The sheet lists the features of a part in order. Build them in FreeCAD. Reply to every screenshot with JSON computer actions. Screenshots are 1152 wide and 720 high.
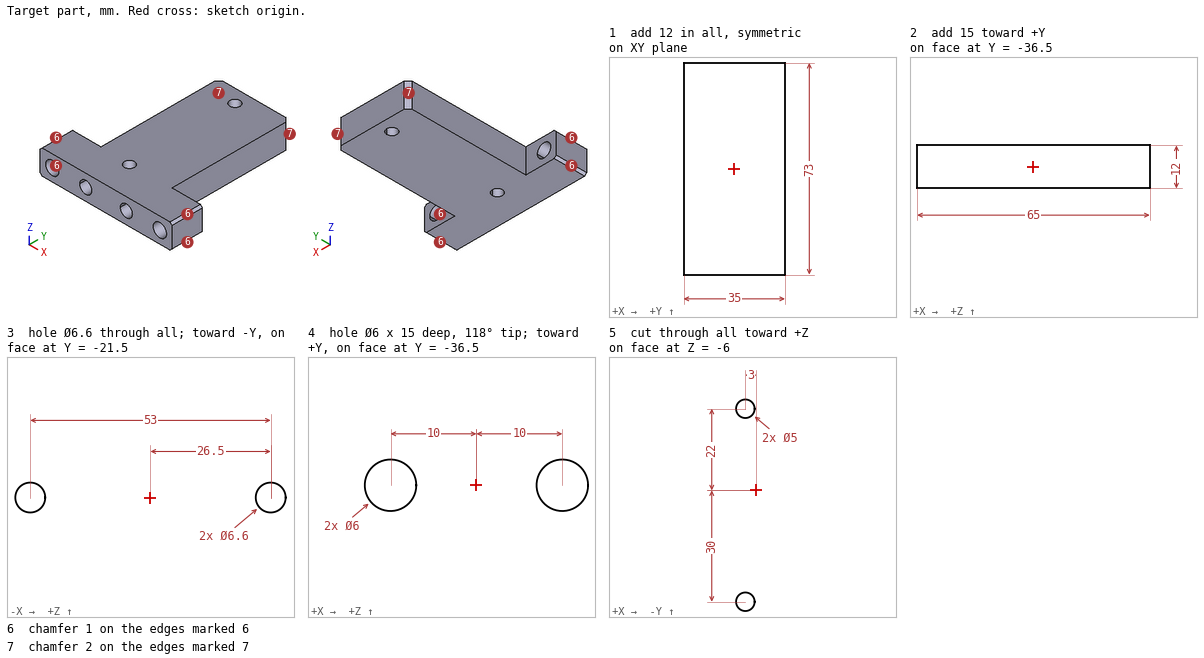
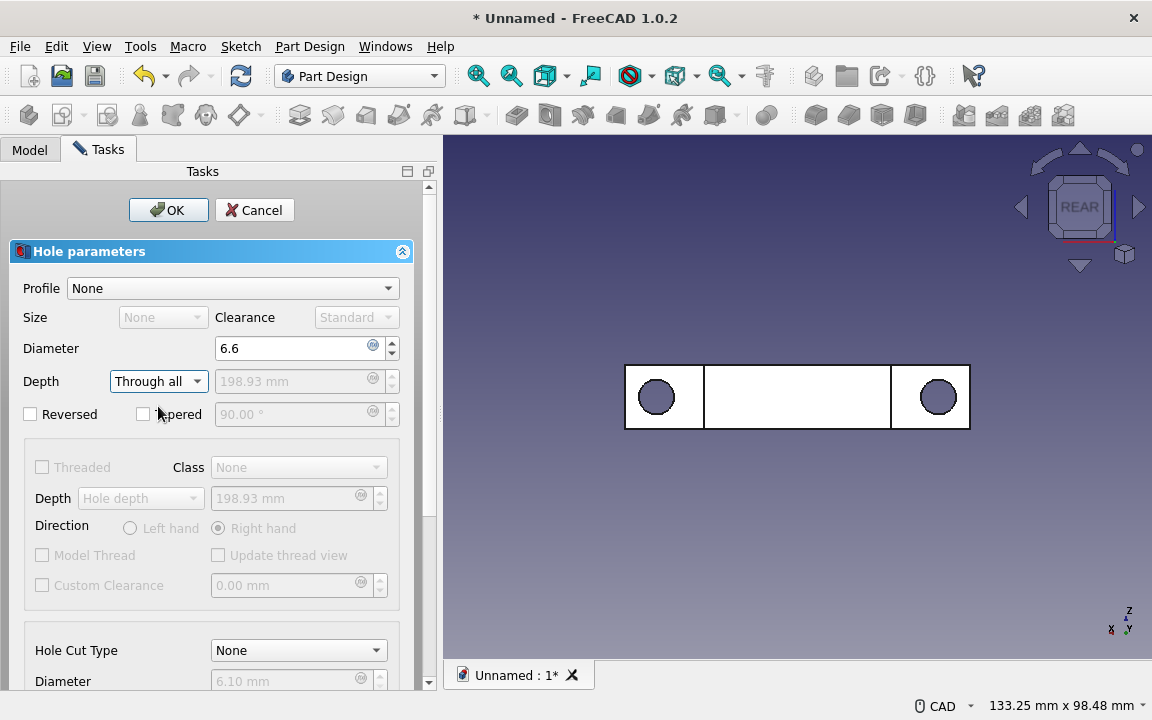
{"action": "left_click", "coordinate": [169, 210]}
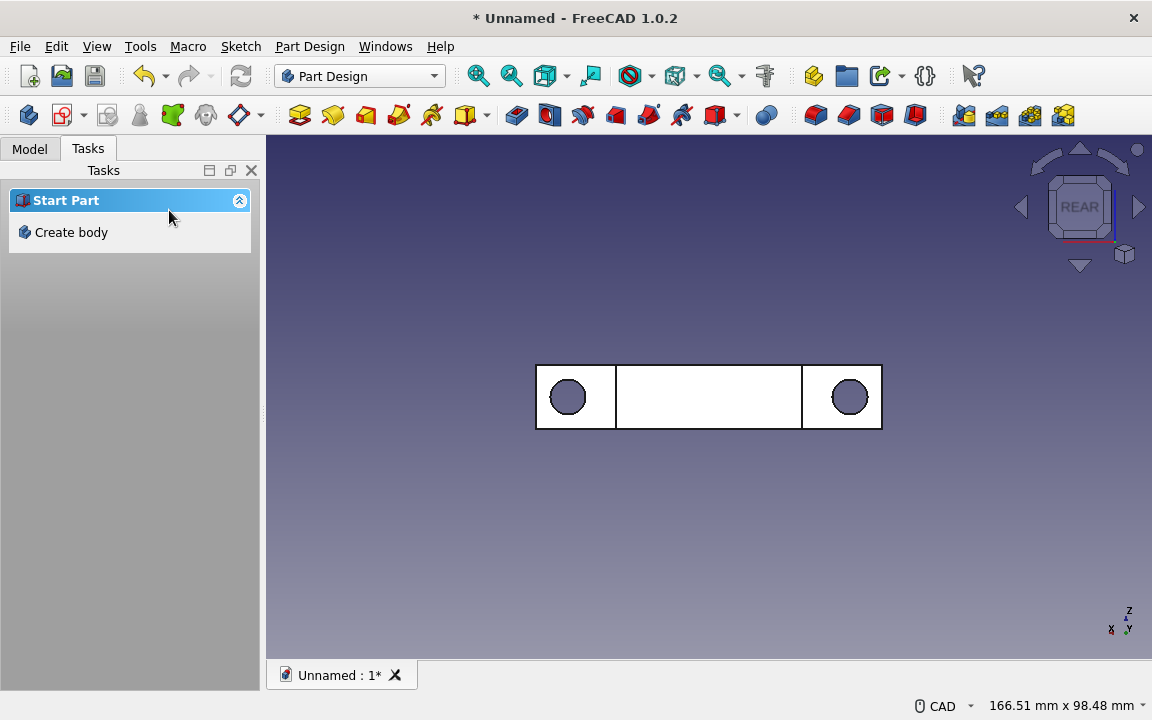
{"action": "left_click", "coordinate": [479, 76]}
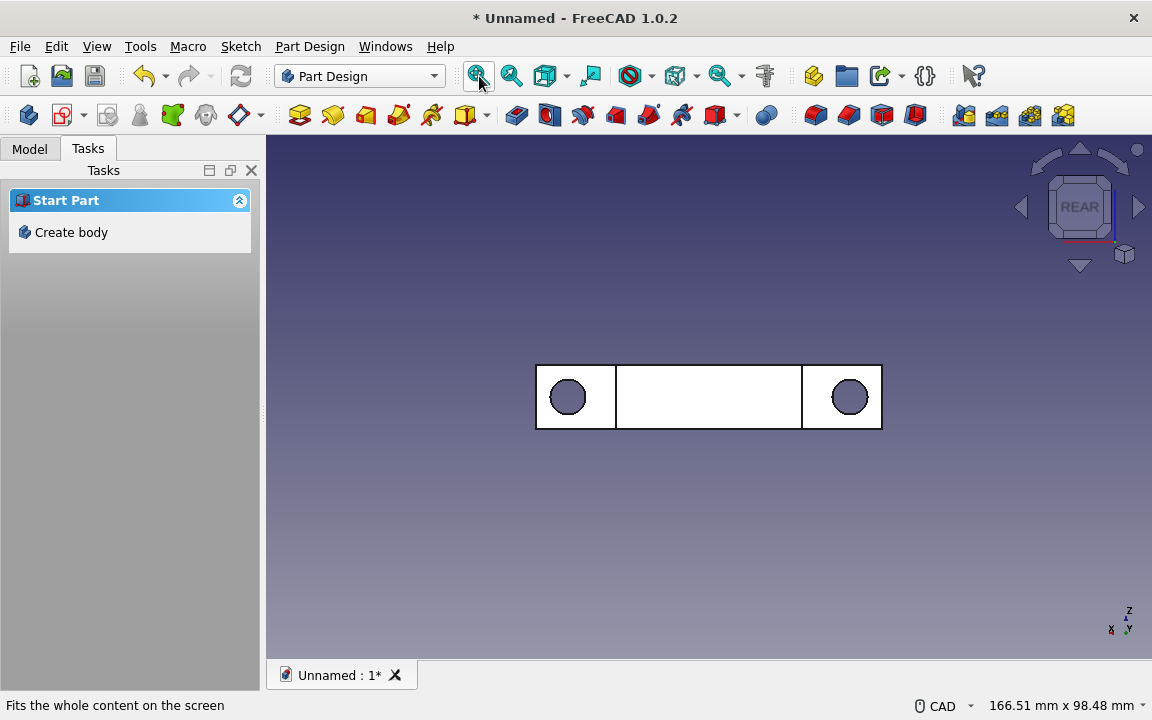
{"action": "key", "text": "0"}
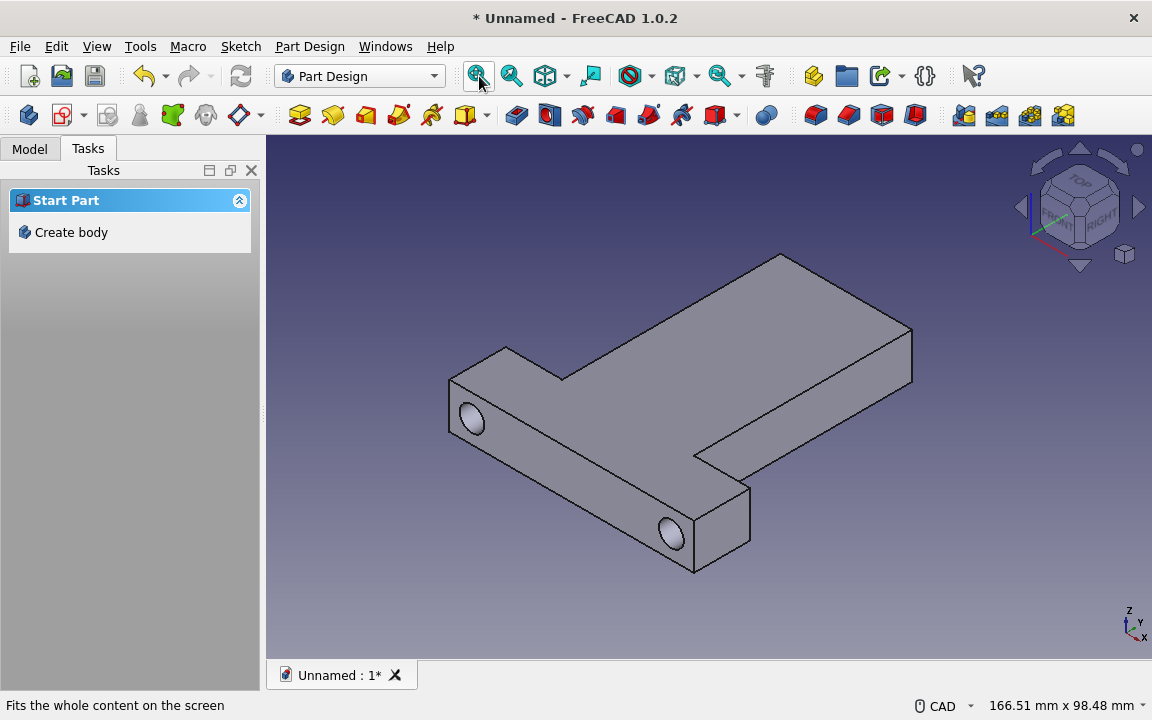
{"action": "left_click", "coordinate": [607, 495]}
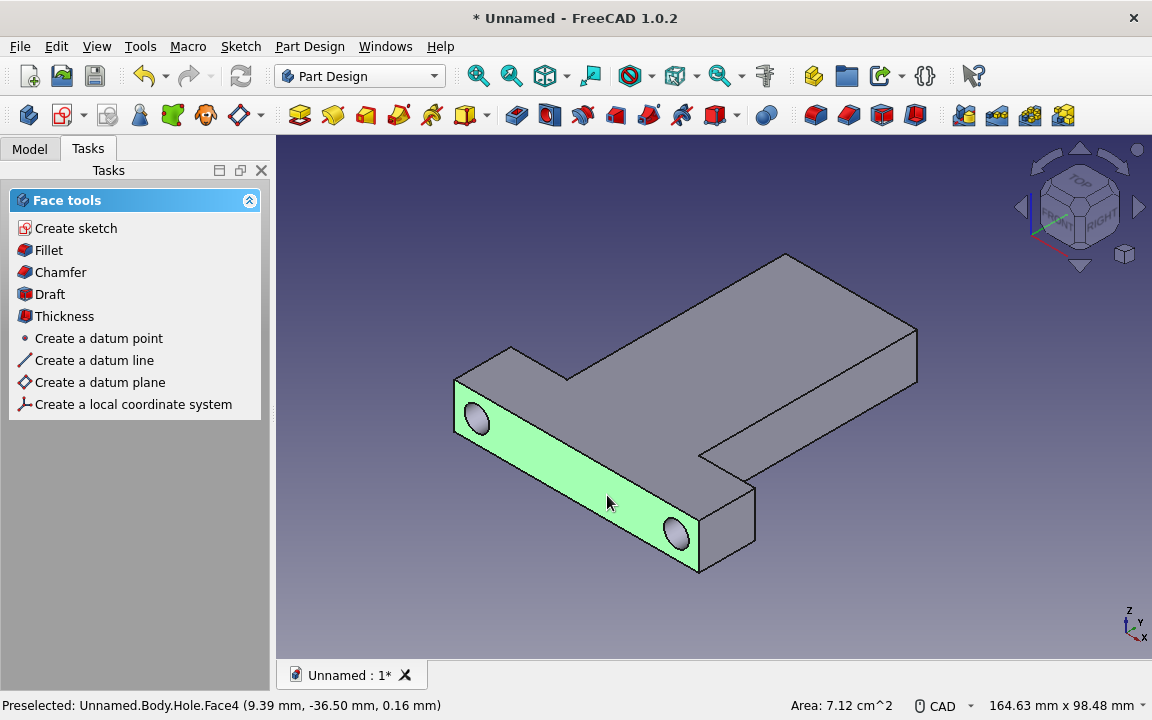
{"action": "left_click", "coordinate": [62, 116]}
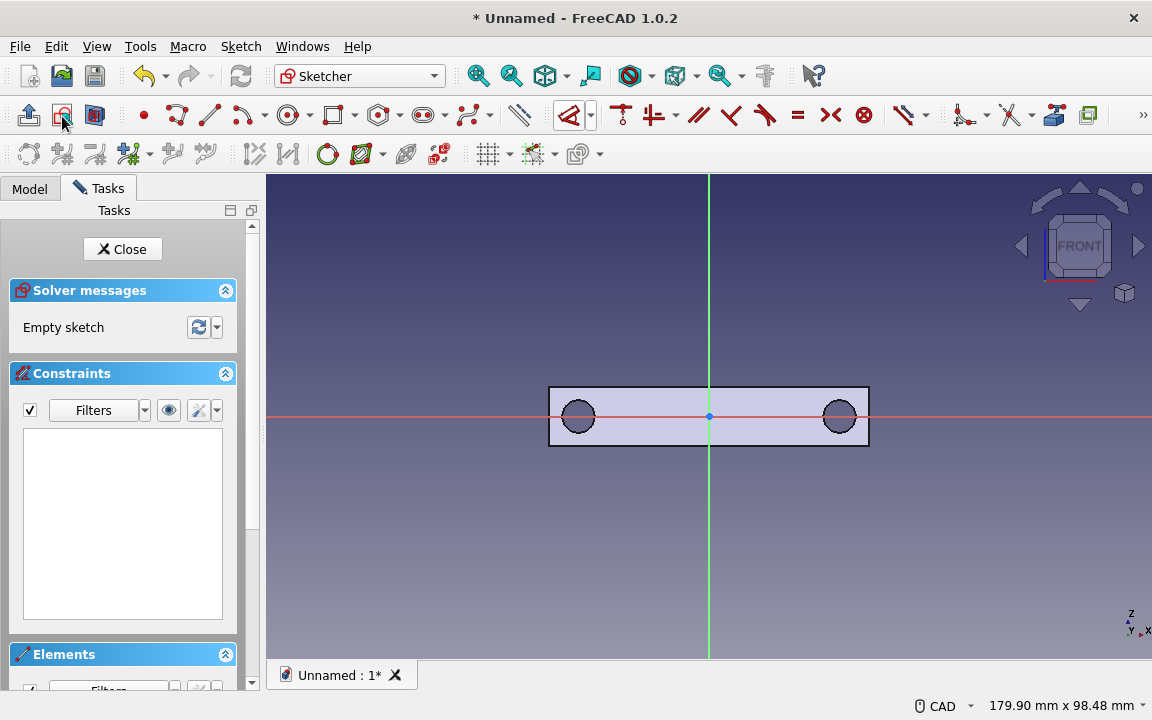
{"action": "scroll", "coordinate": [731, 417], "scroll_direction": "up", "scroll_amount": 7}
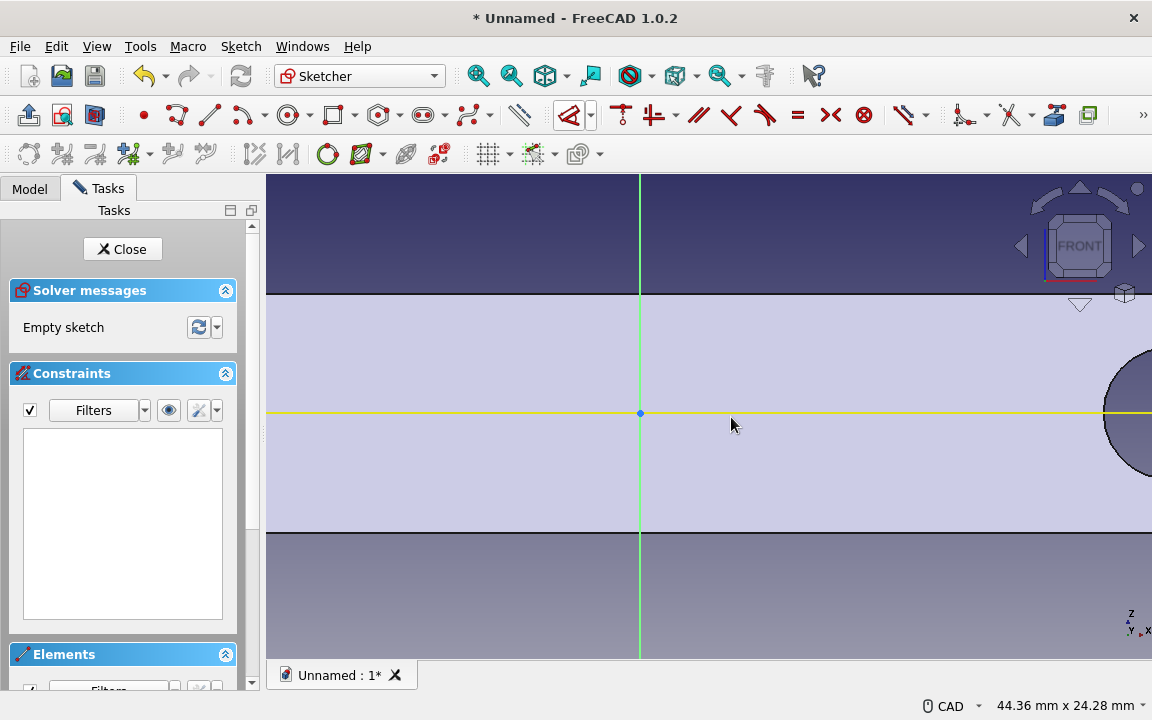
{"action": "left_click", "coordinate": [288, 116]}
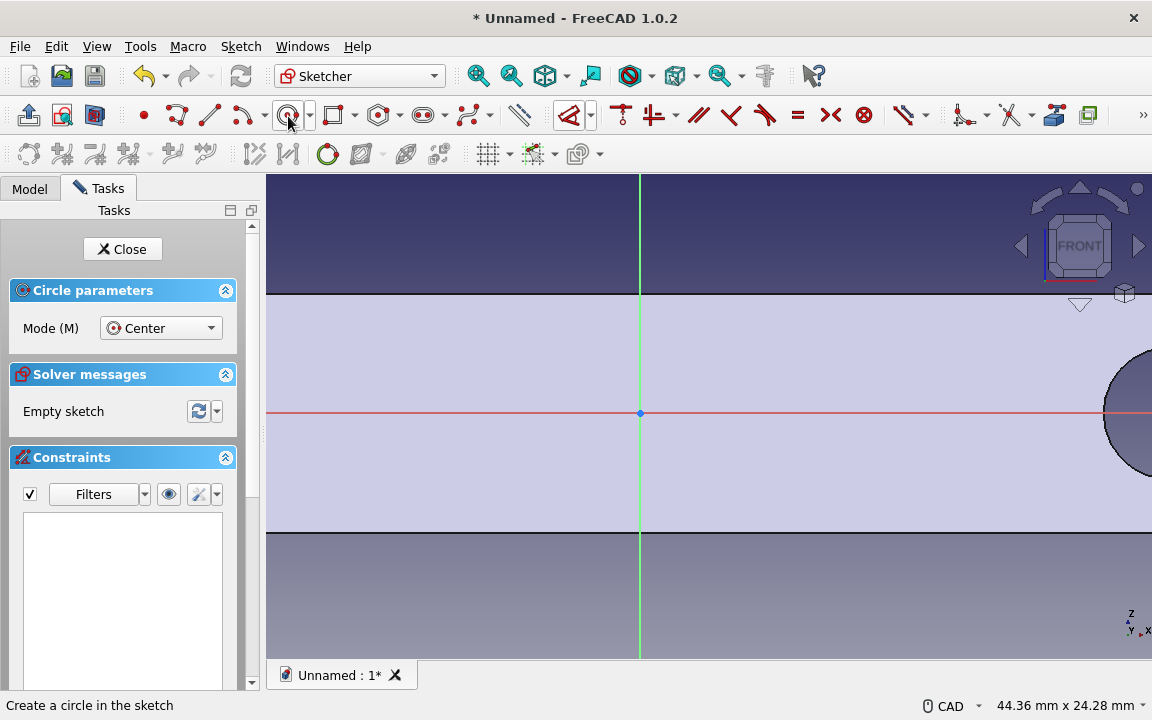
{"action": "left_click", "coordinate": [440, 413]}
{"action": "mouse_move", "coordinate": [483, 371]}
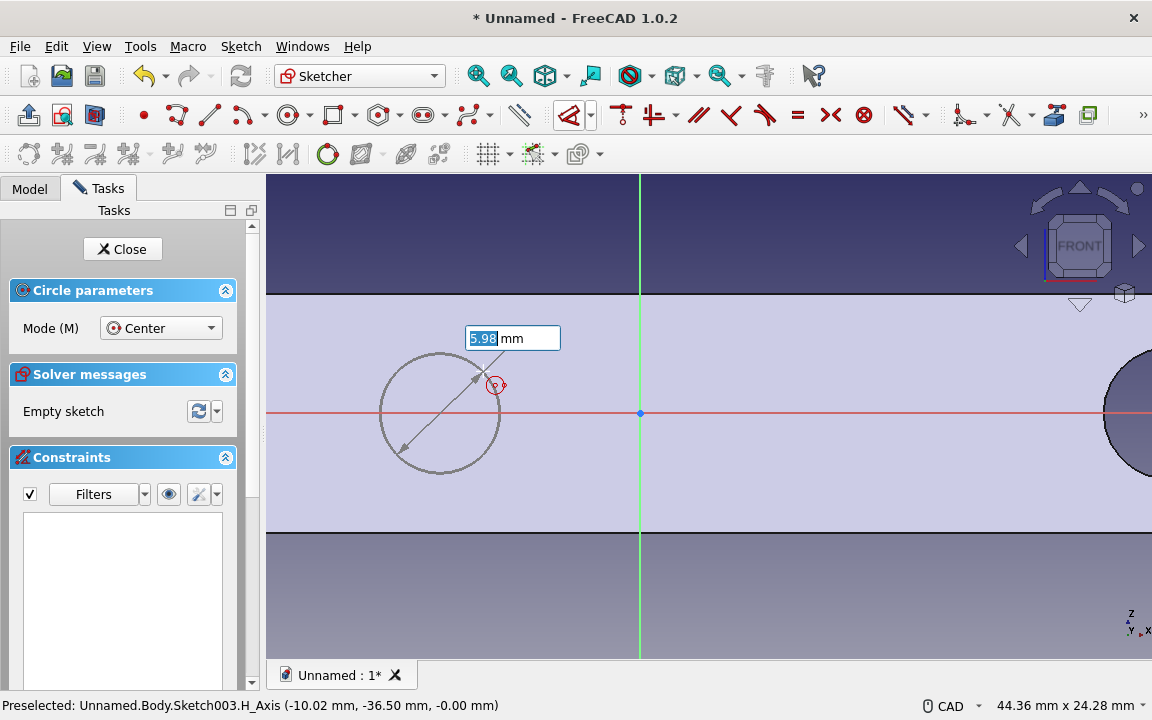
{"action": "type", "text": "6"}
{"action": "key", "text": "Return"}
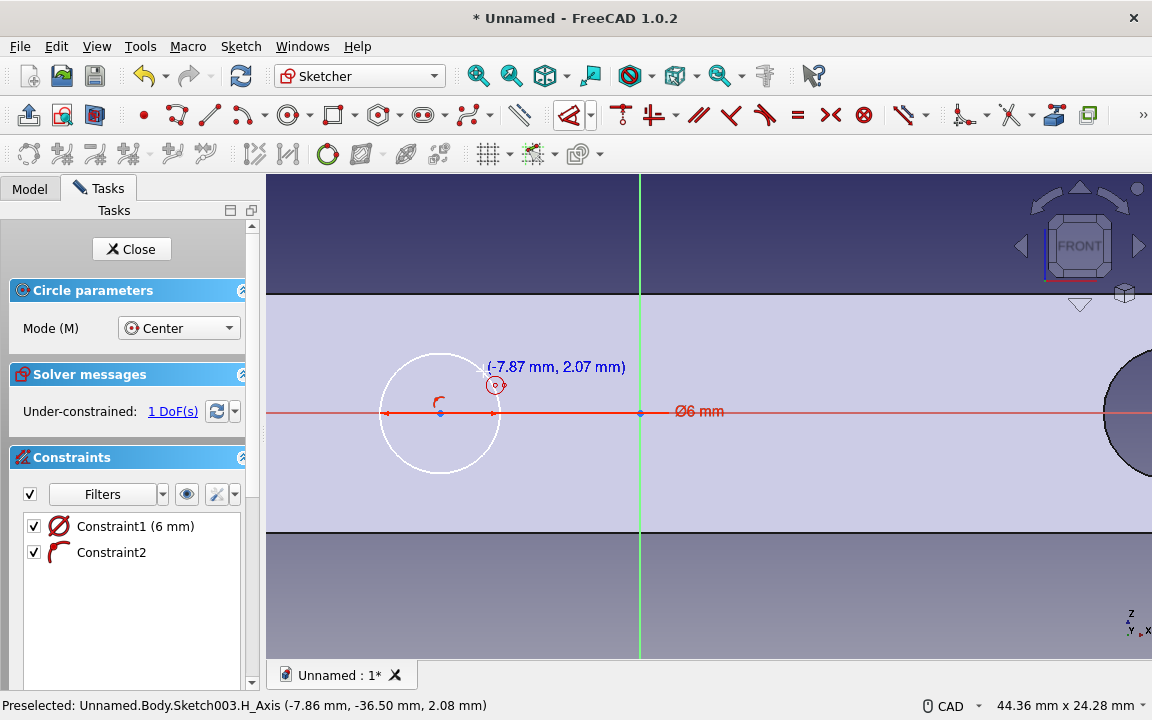
{"action": "left_click", "coordinate": [840, 413]}
{"action": "mouse_move", "coordinate": [882, 371]}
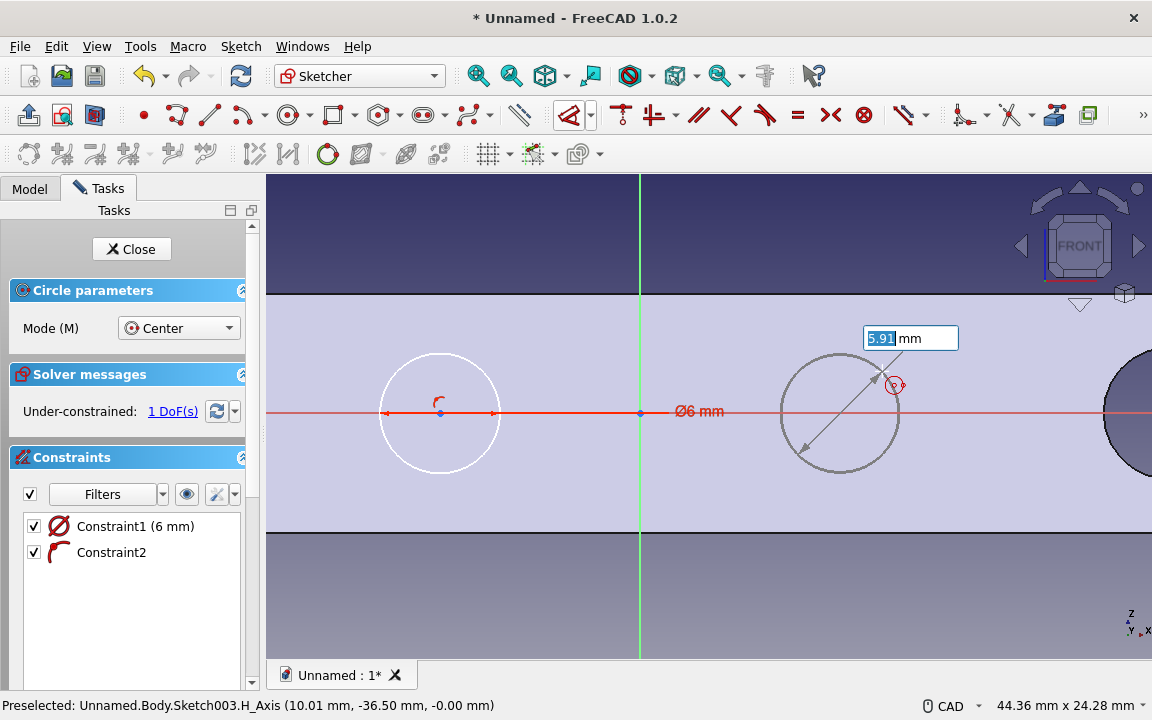
{"action": "type", "text": "6"}
{"action": "key", "text": "Return"}
{"action": "key", "text": "Escape"}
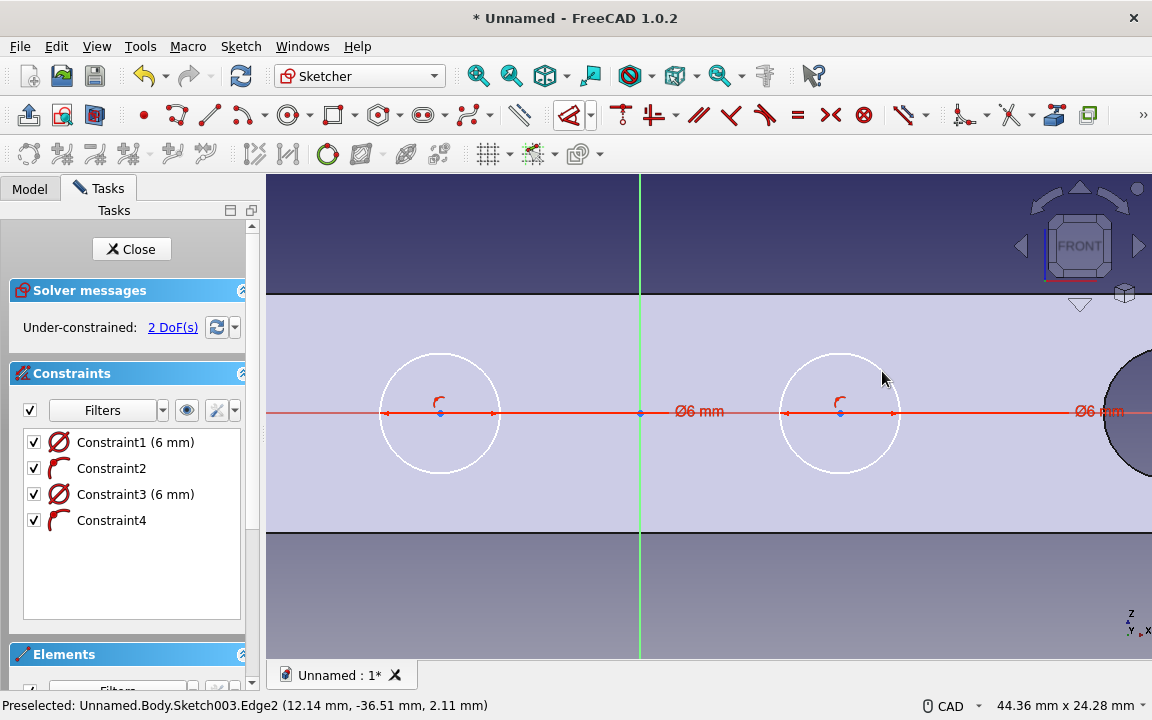
{"action": "left_click", "coordinate": [440, 413]}